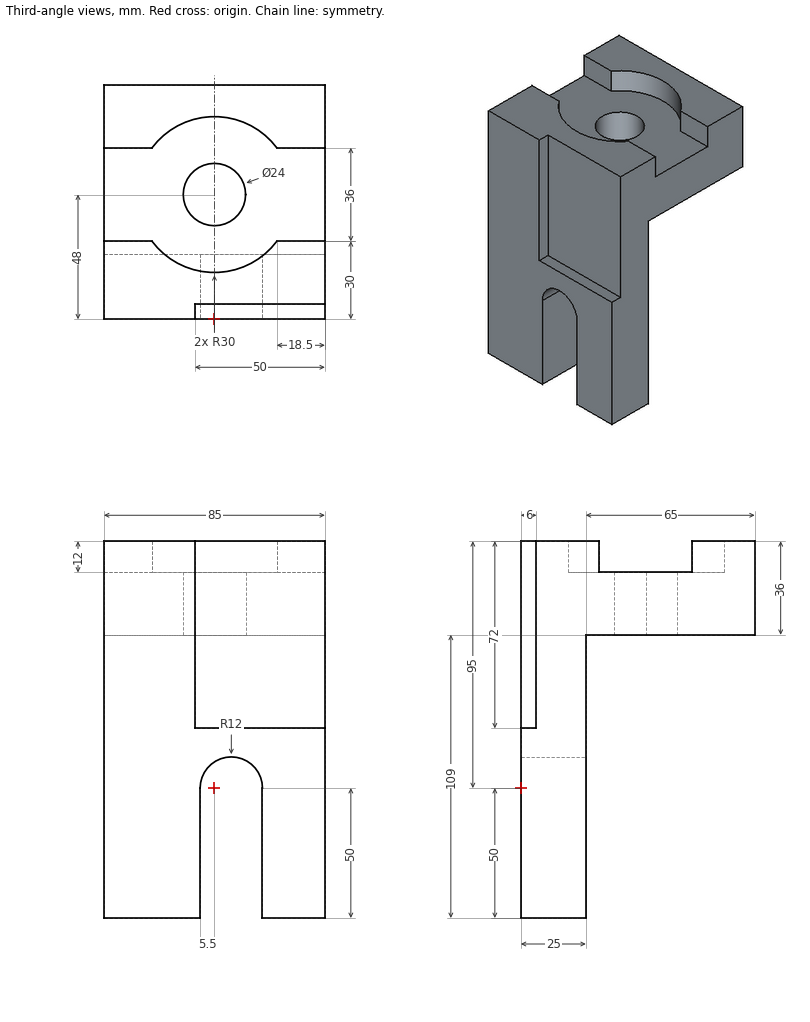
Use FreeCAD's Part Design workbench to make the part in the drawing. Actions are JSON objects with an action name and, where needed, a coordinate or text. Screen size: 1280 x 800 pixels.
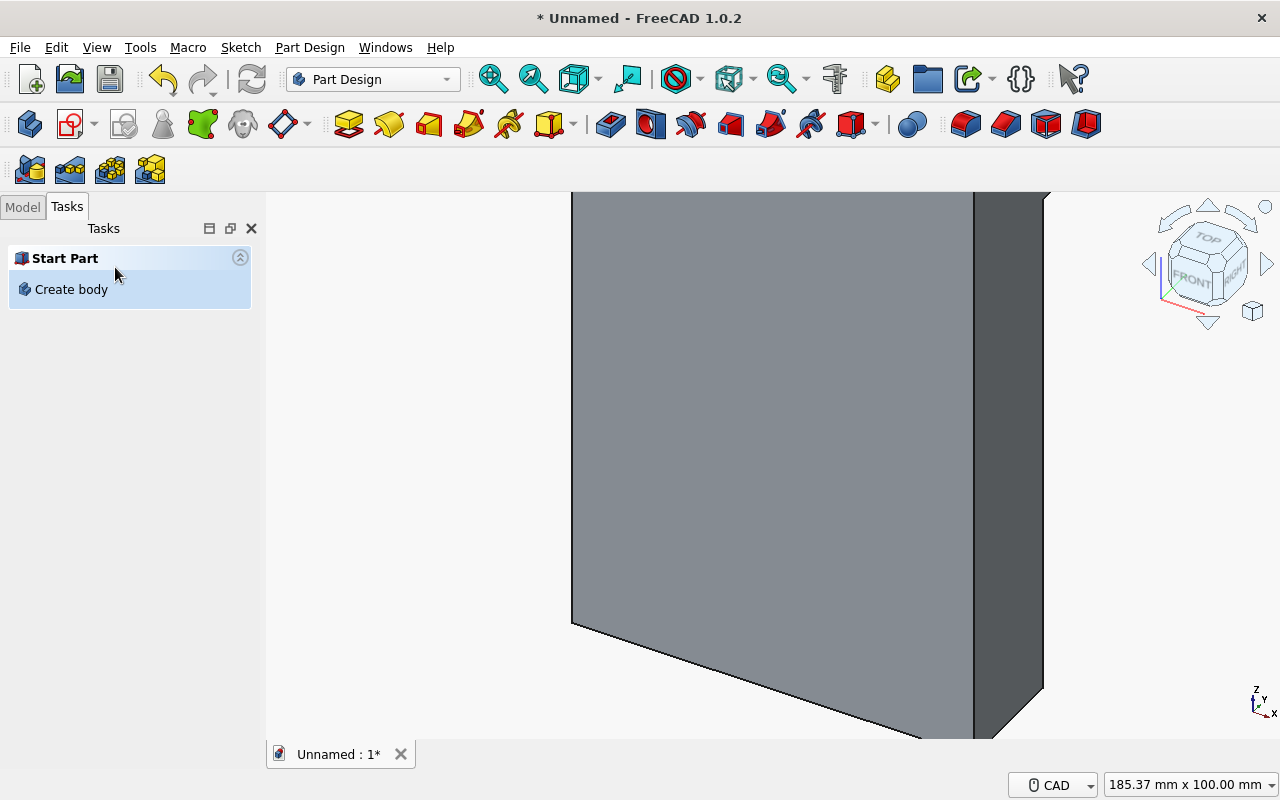
{"action": "left_click", "coordinate": [494, 80]}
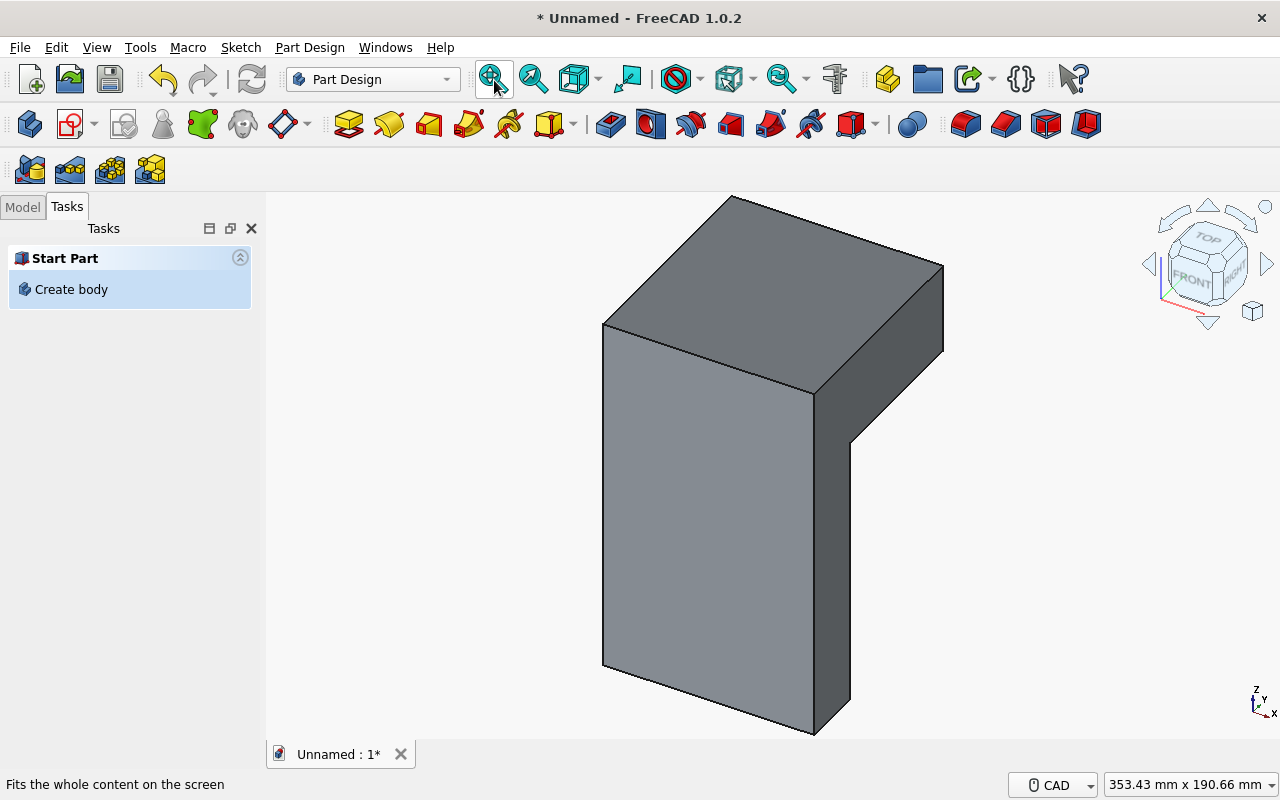
{"action": "key", "text": "4"}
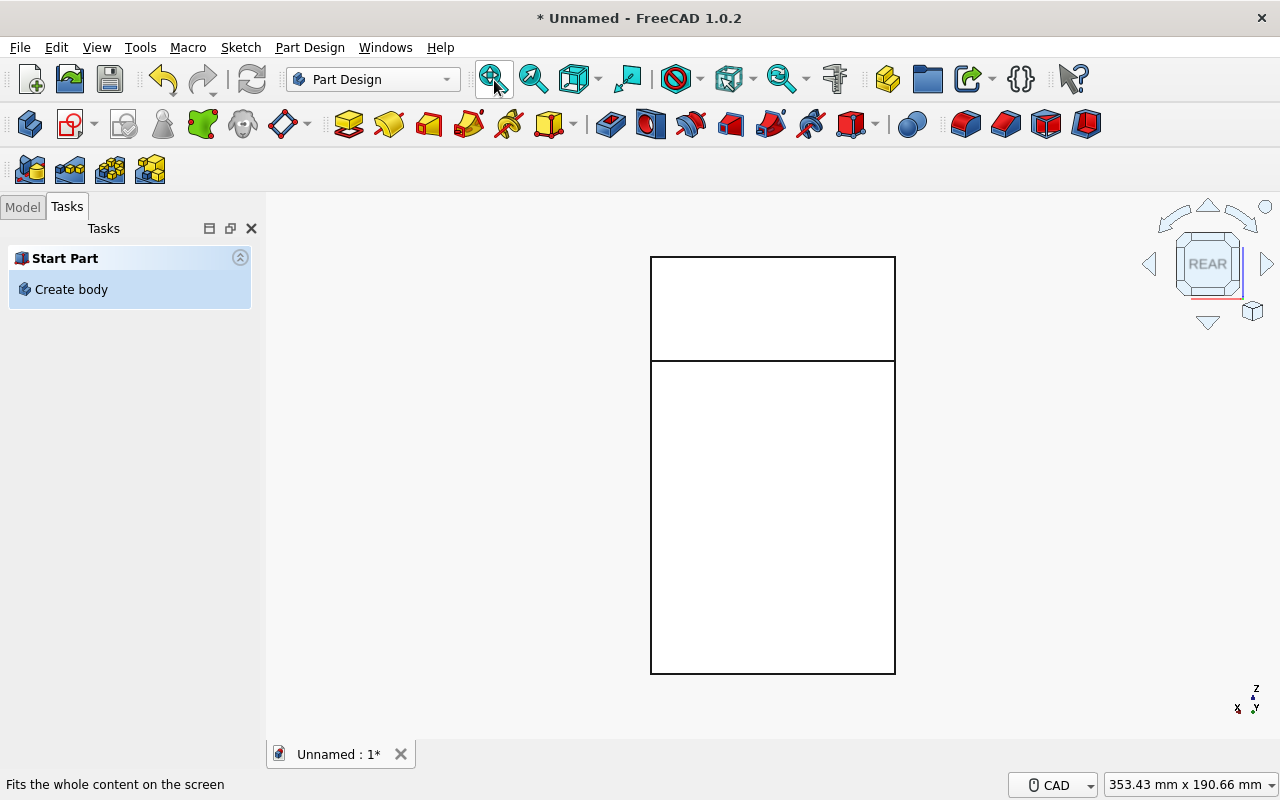
{"action": "left_click", "coordinate": [773, 516]}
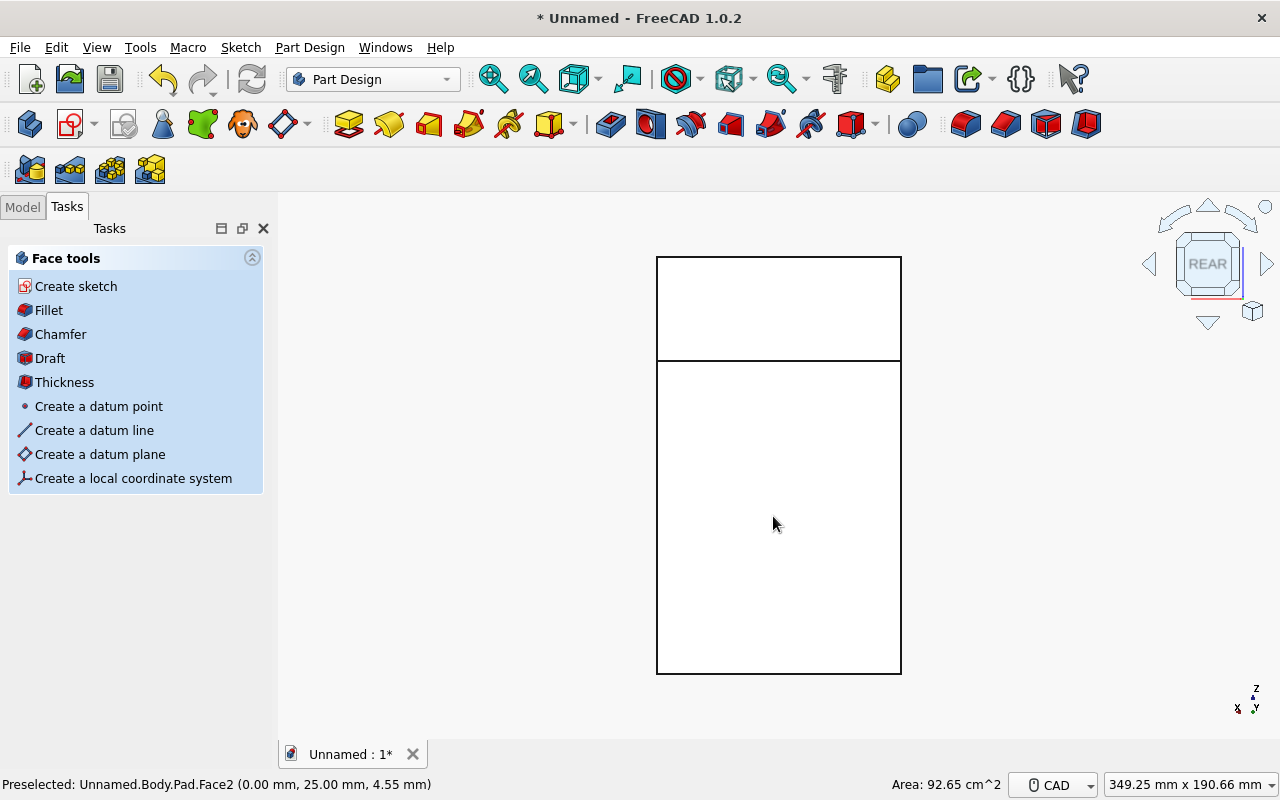
{"action": "left_click", "coordinate": [70, 124]}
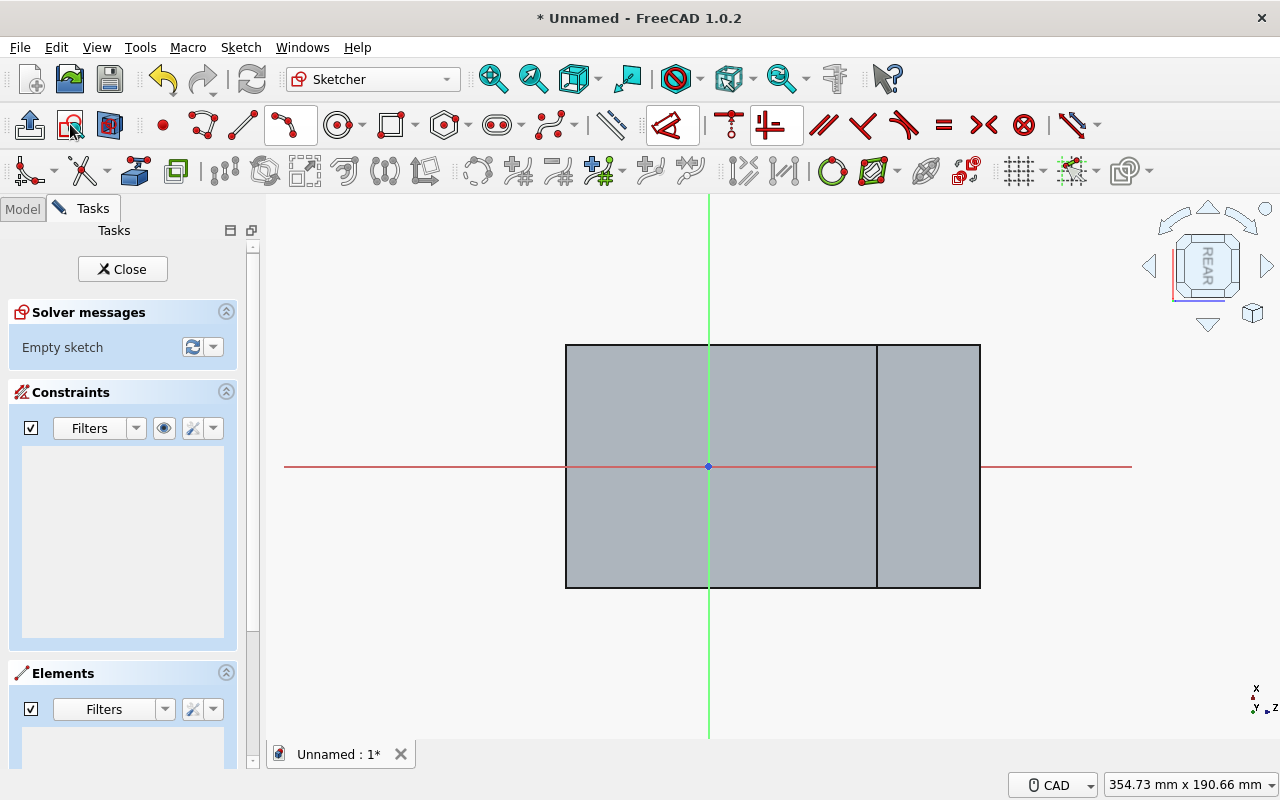
{"action": "left_click", "coordinate": [110, 126]}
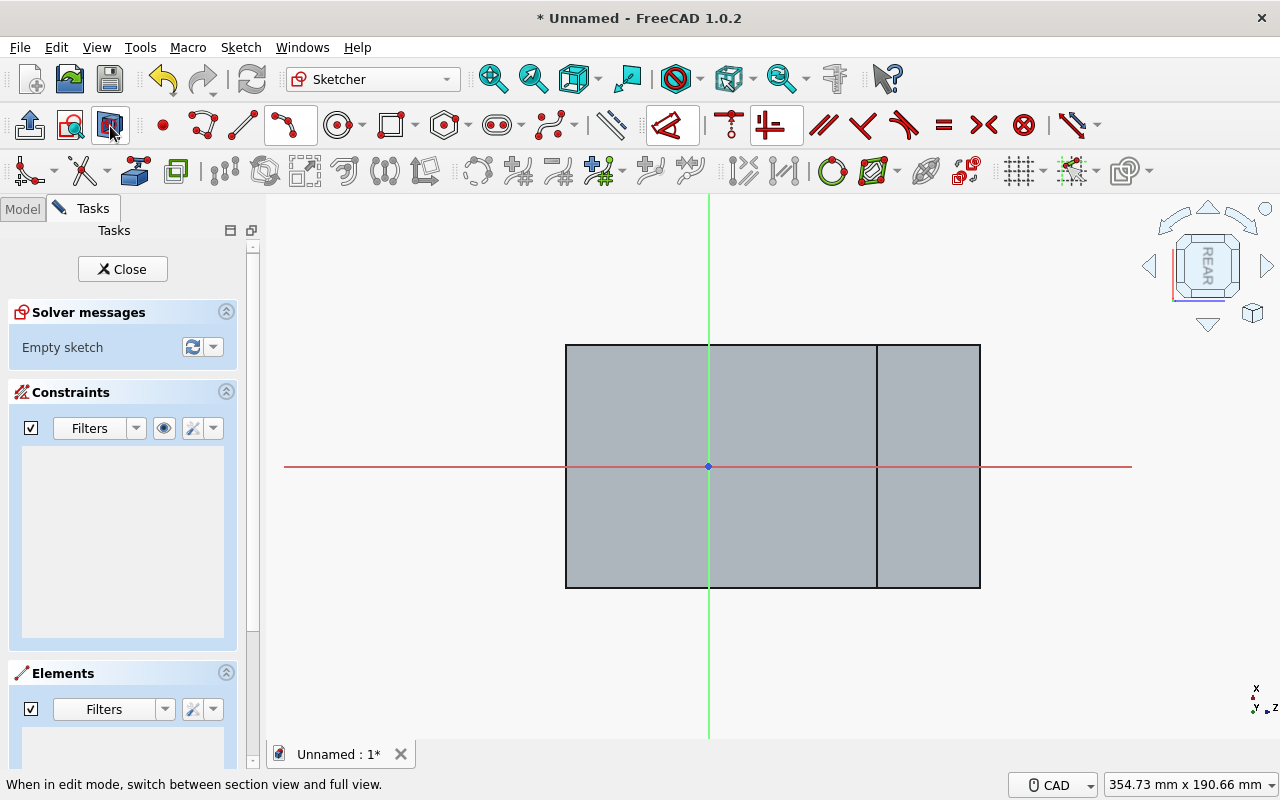
{"action": "scroll", "coordinate": [633, 440], "scroll_direction": "up", "scroll_amount": 6}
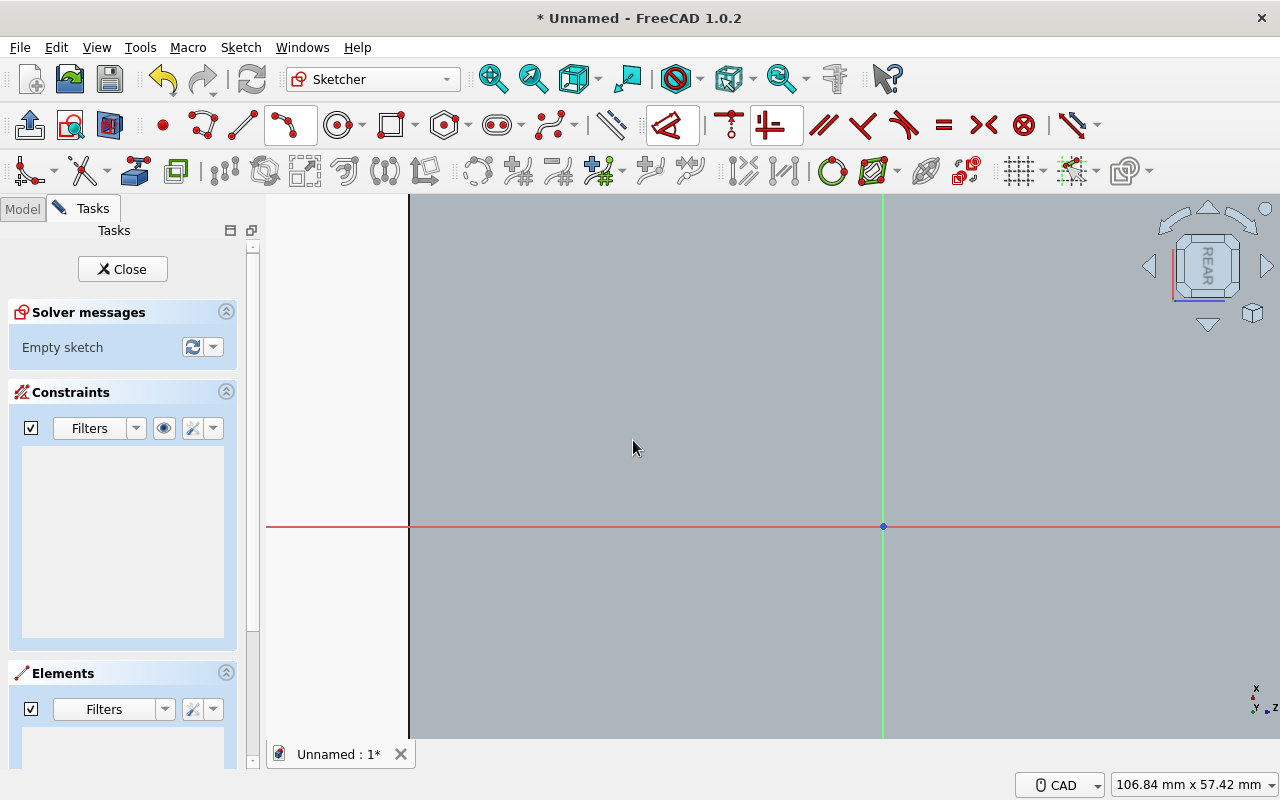
{"action": "left_click", "coordinate": [204, 126]}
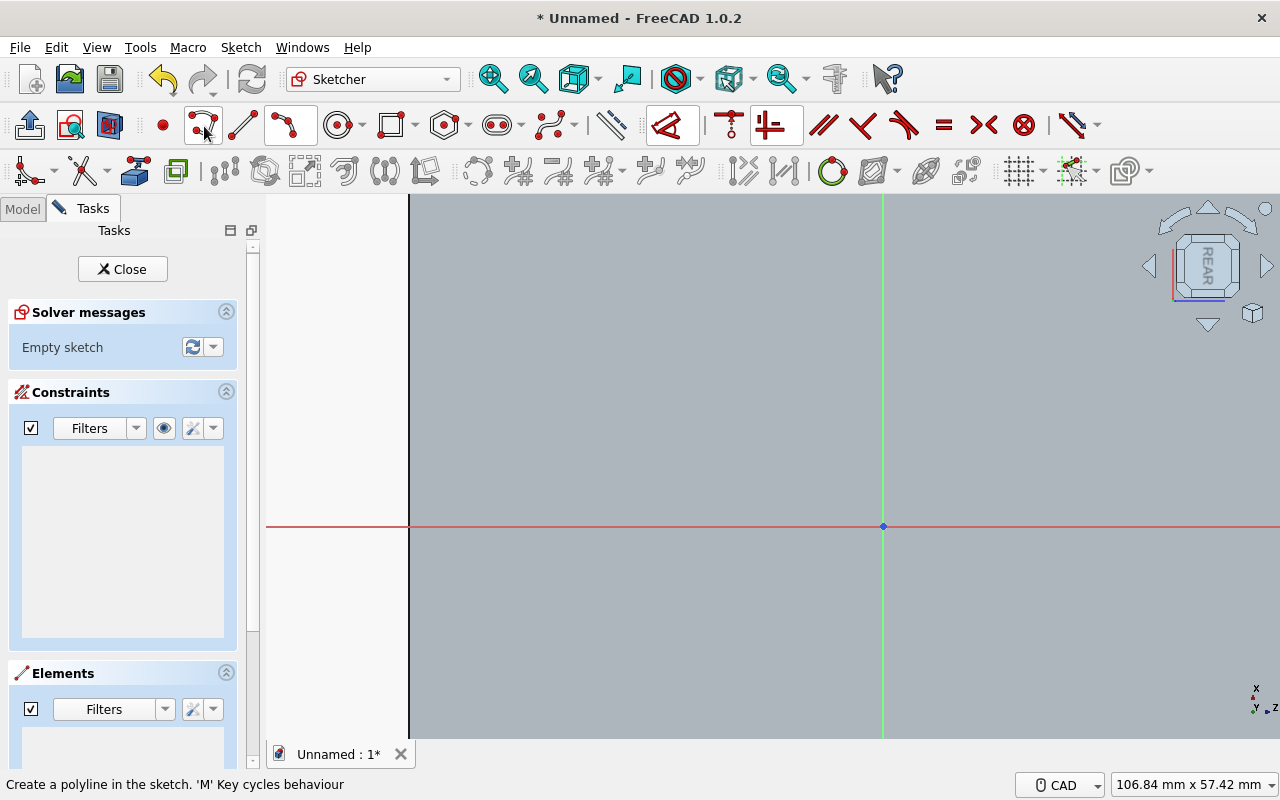
{"action": "left_click", "coordinate": [883, 351]}
{"action": "left_click", "coordinate": [409, 351]}
{"action": "left_click", "coordinate": [409, 579]}
{"action": "left_click", "coordinate": [883, 579]}
{"action": "right_click", "coordinate": [883, 579]}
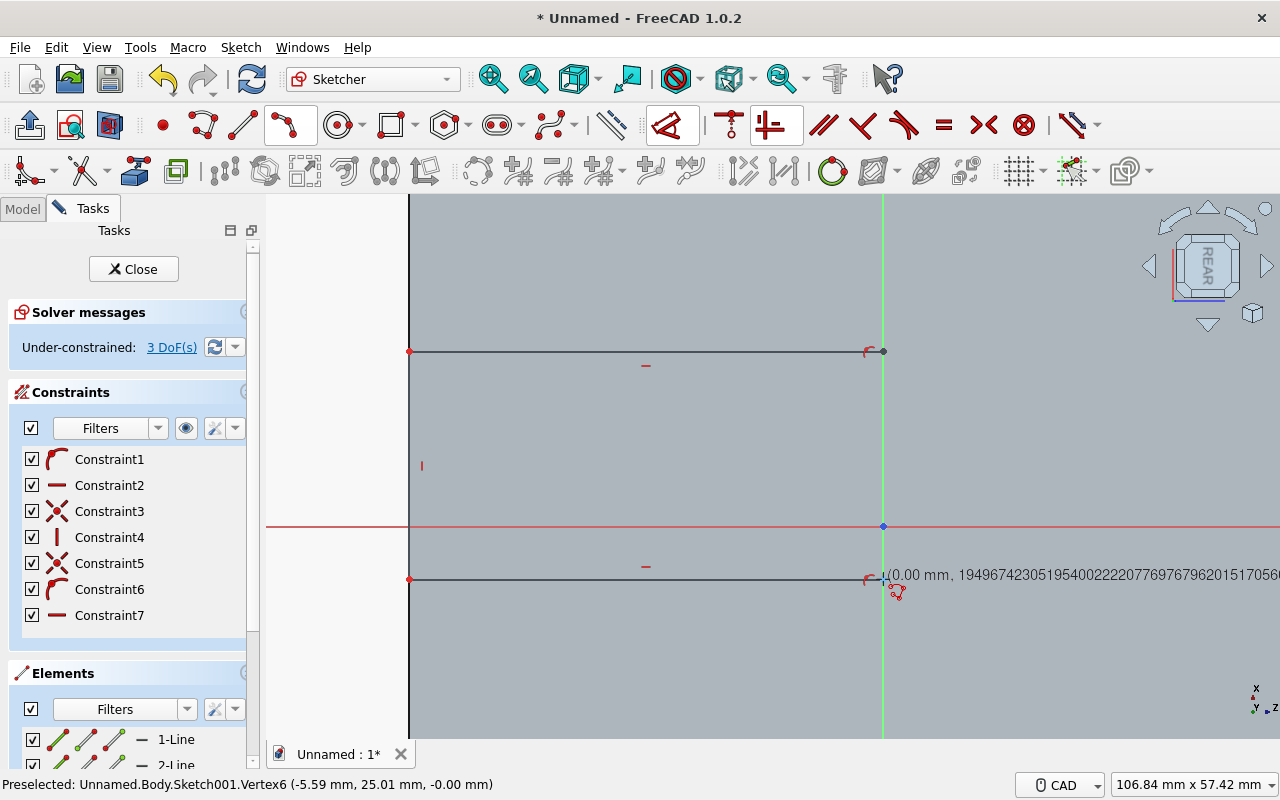
{"action": "left_click", "coordinate": [284, 126]}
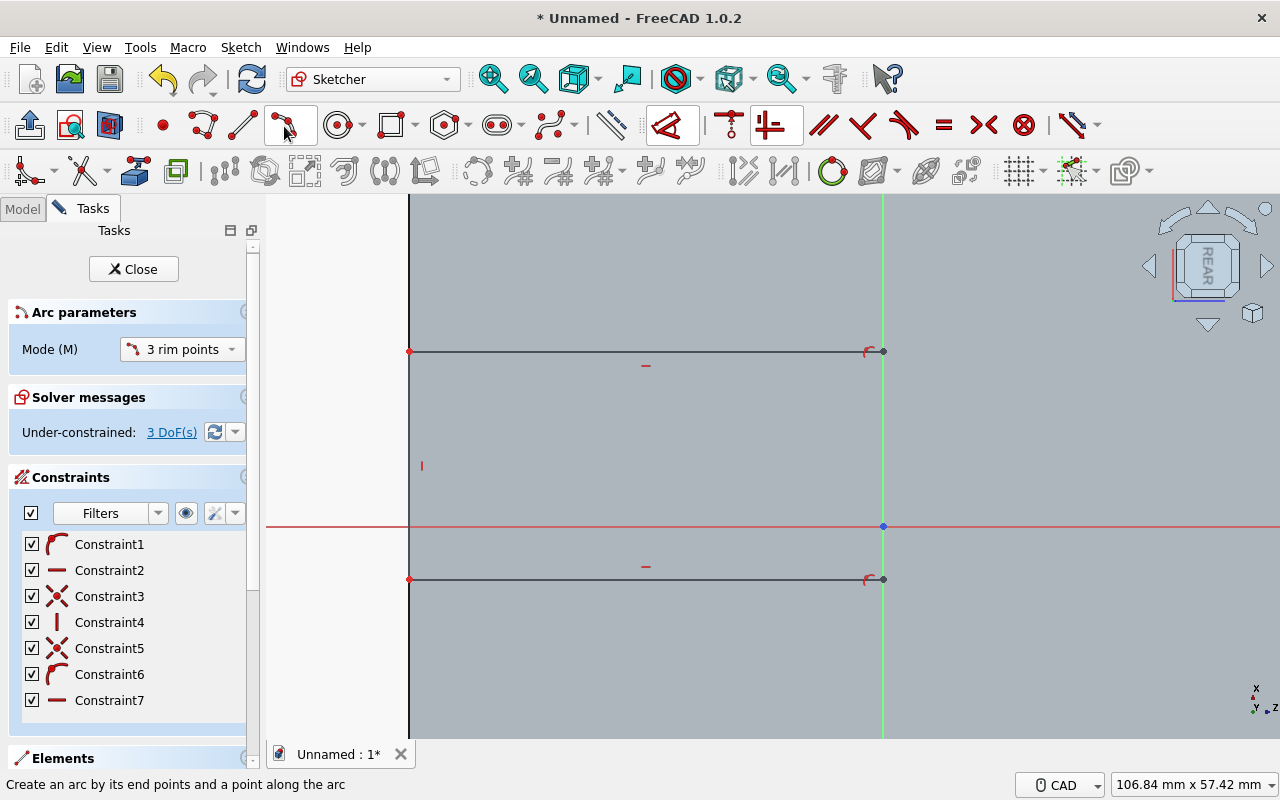
{"action": "left_click", "coordinate": [883, 580]}
{"action": "left_click", "coordinate": [883, 352]}
{"action": "left_click", "coordinate": [997, 465]}
{"action": "key", "text": "Escape"}